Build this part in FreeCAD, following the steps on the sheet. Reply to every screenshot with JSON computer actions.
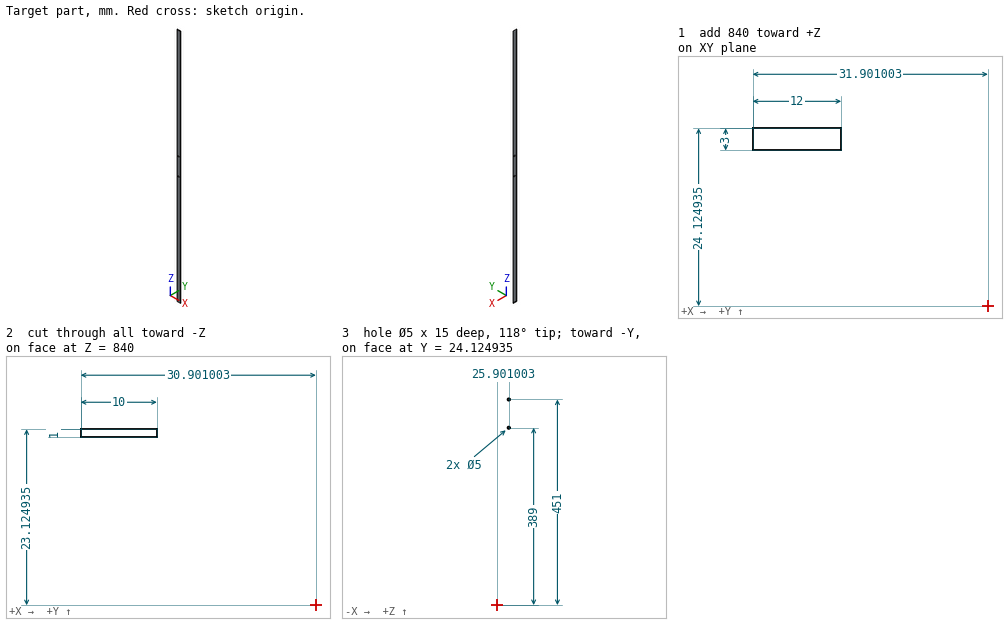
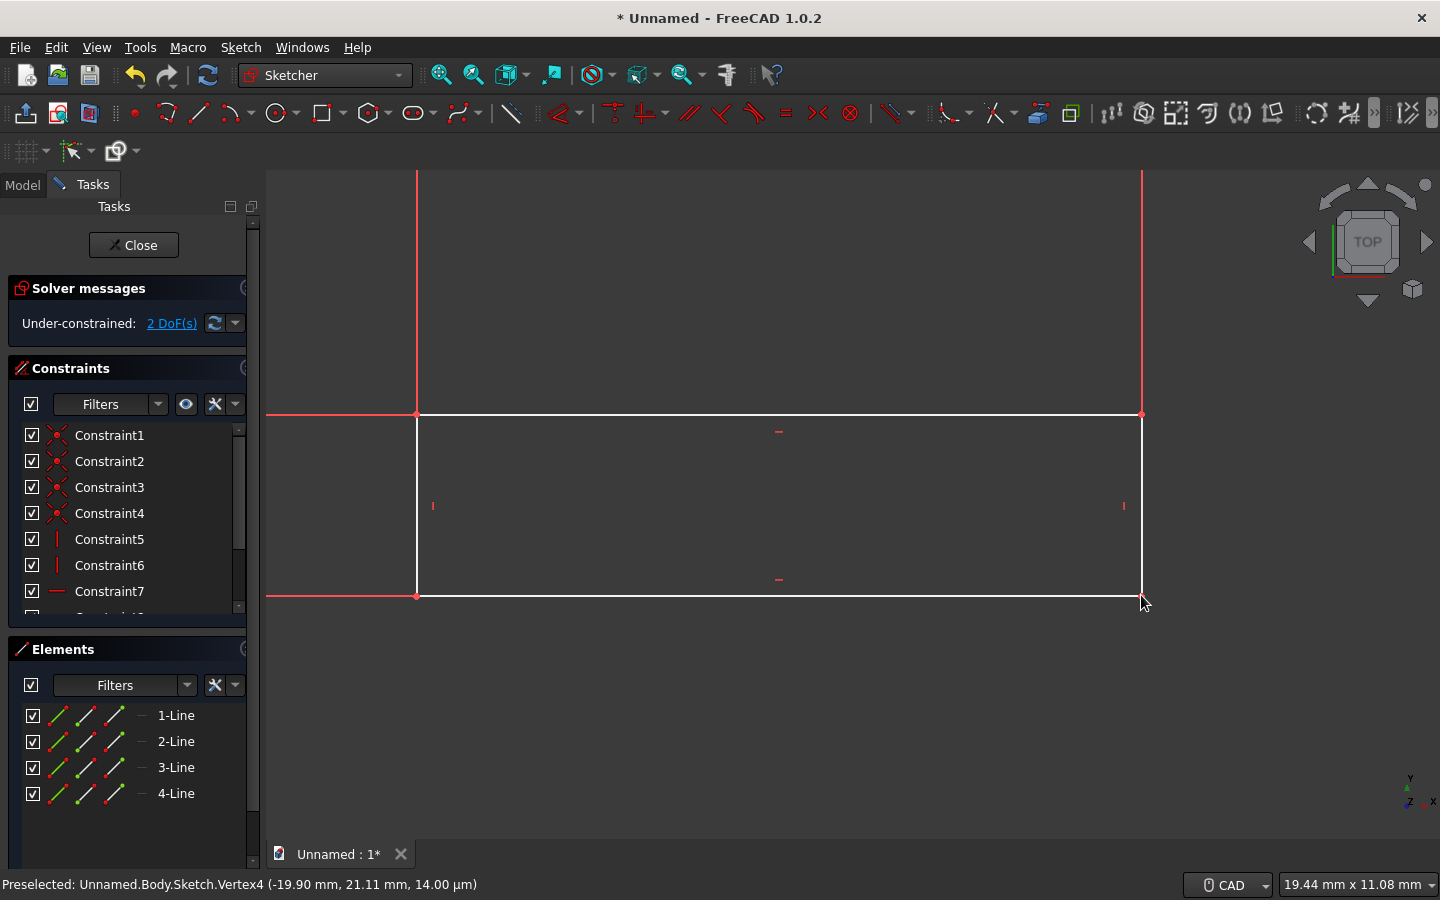
{"action": "left_click", "coordinate": [558, 114]}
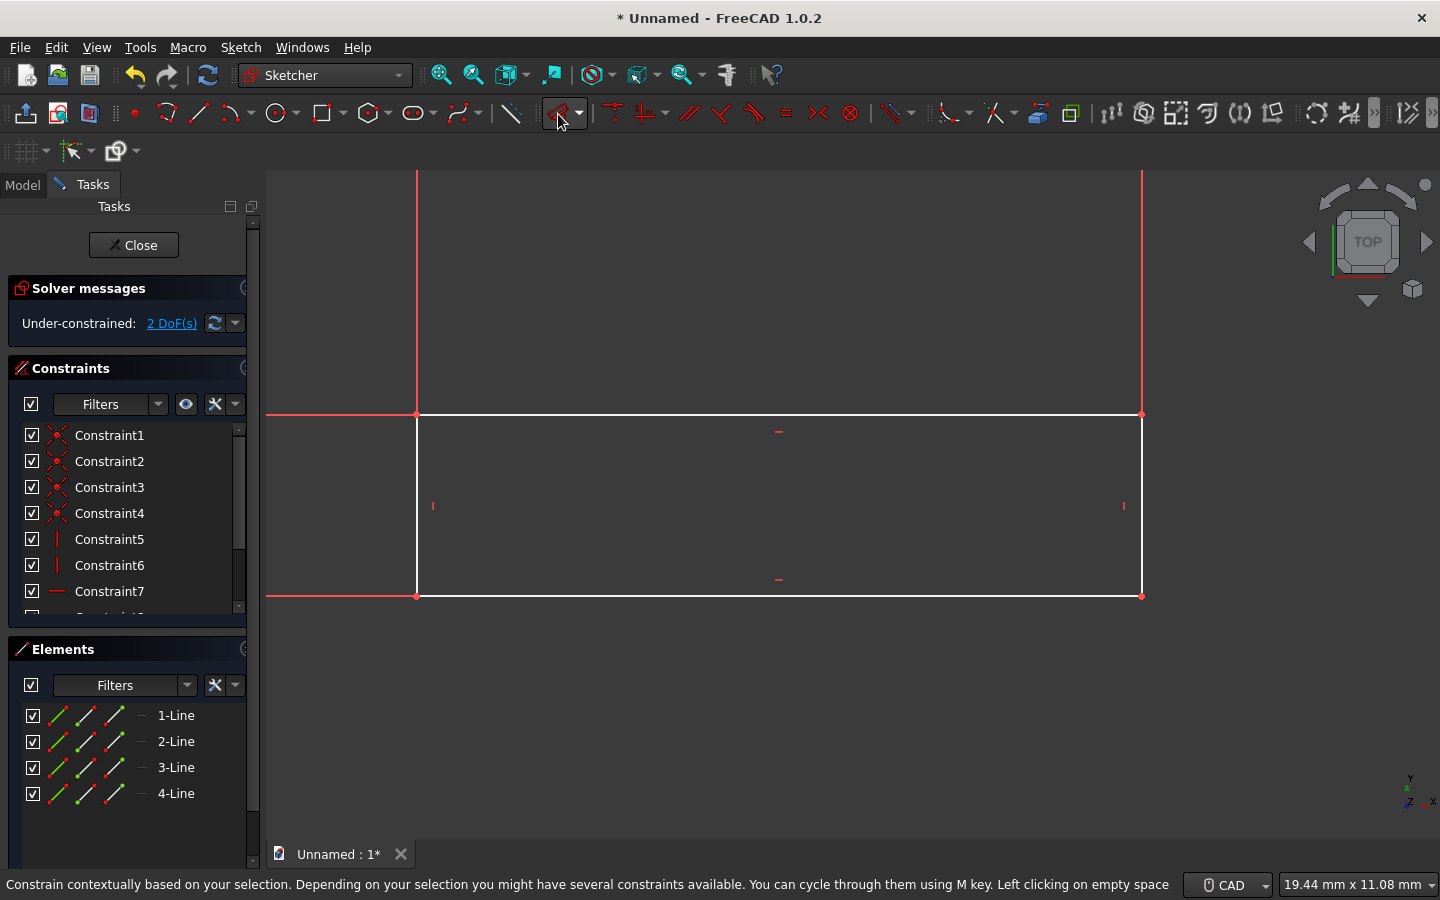
{"action": "left_click", "coordinate": [417, 415]}
{"action": "left_click", "coordinate": [846, 381]}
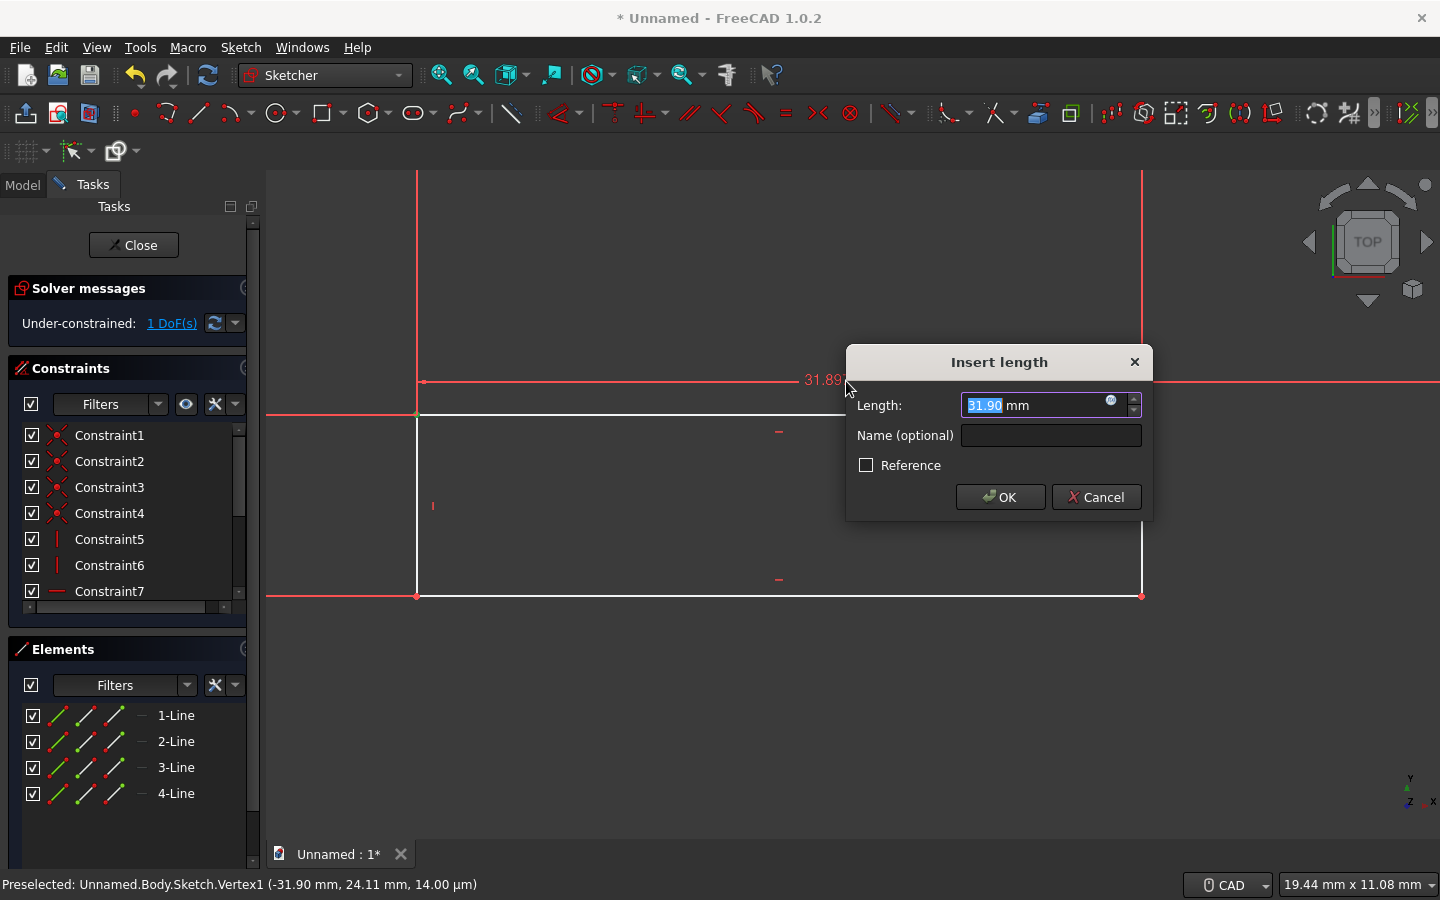
{"action": "type", "text": "31.901003"}
{"action": "key", "text": "Return"}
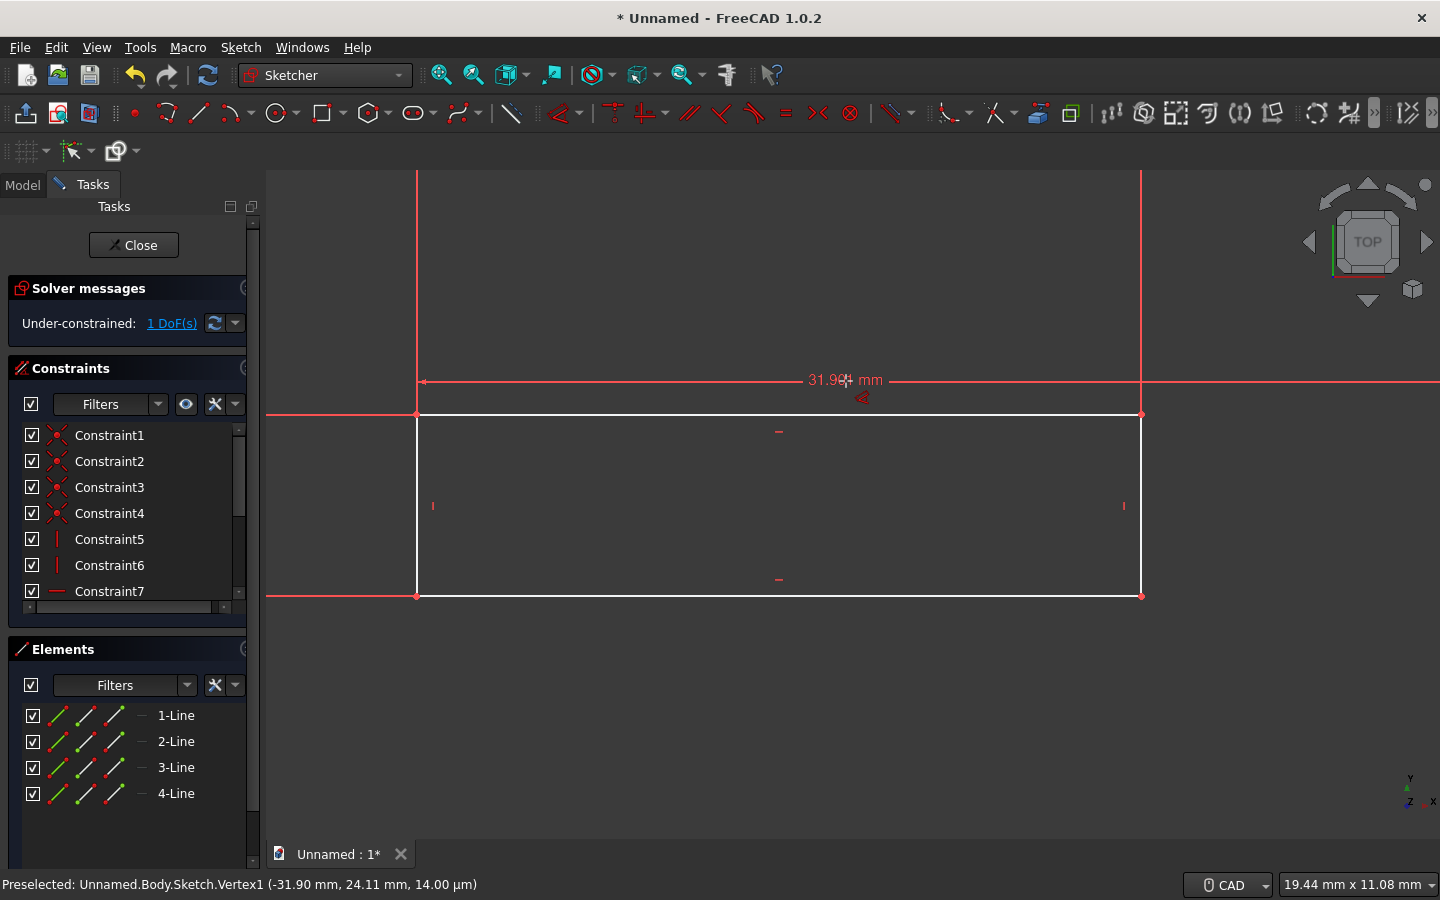
{"action": "left_click", "coordinate": [417, 415]}
{"action": "left_click", "coordinate": [383, 613]}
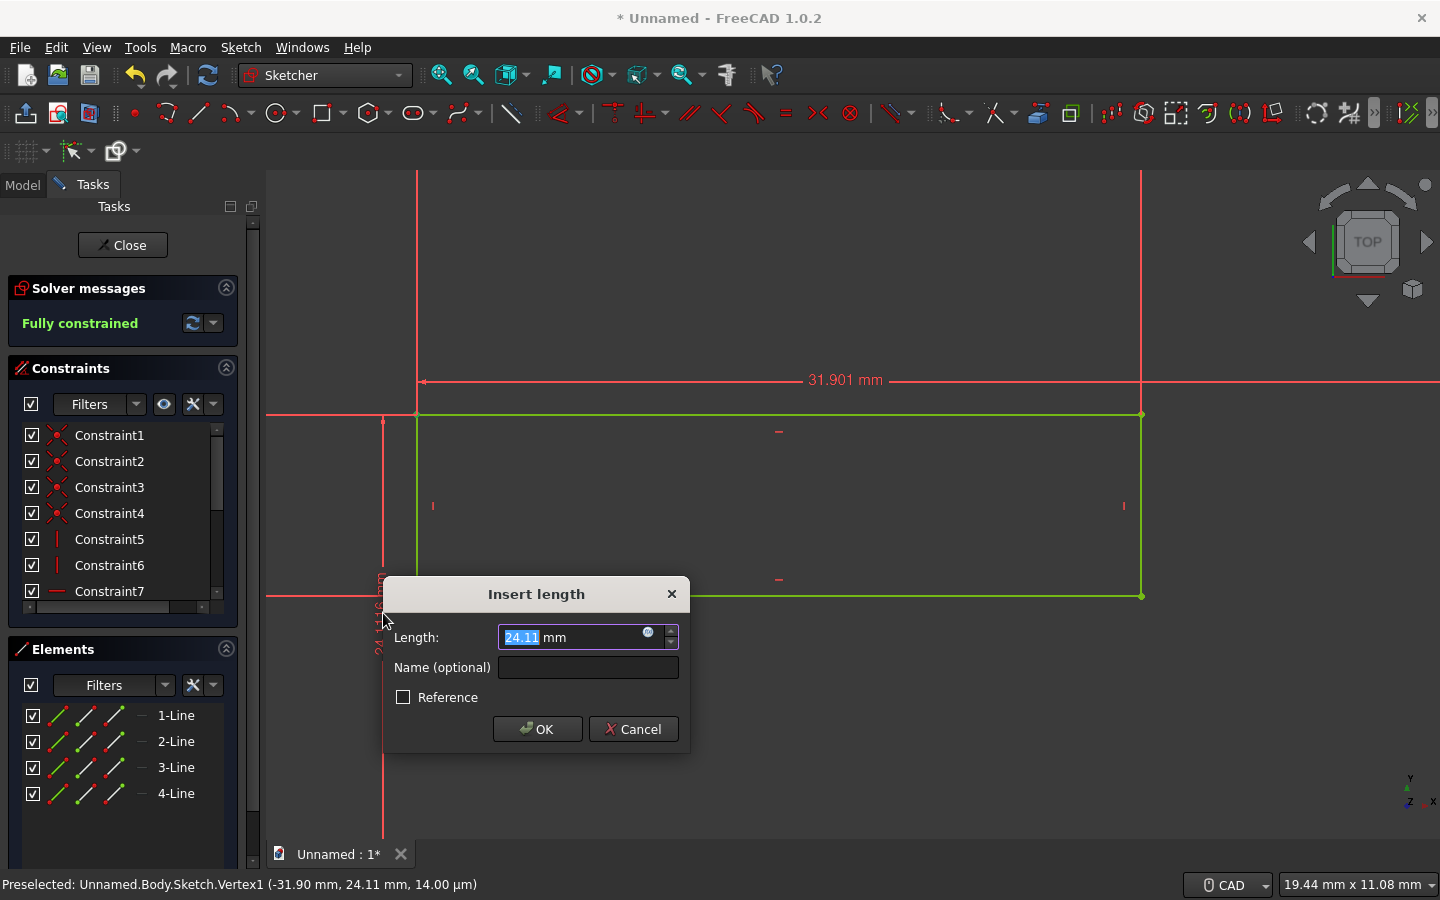
{"action": "type", "text": "24.124935"}
{"action": "key", "text": "Return"}
{"action": "key", "text": "Escape"}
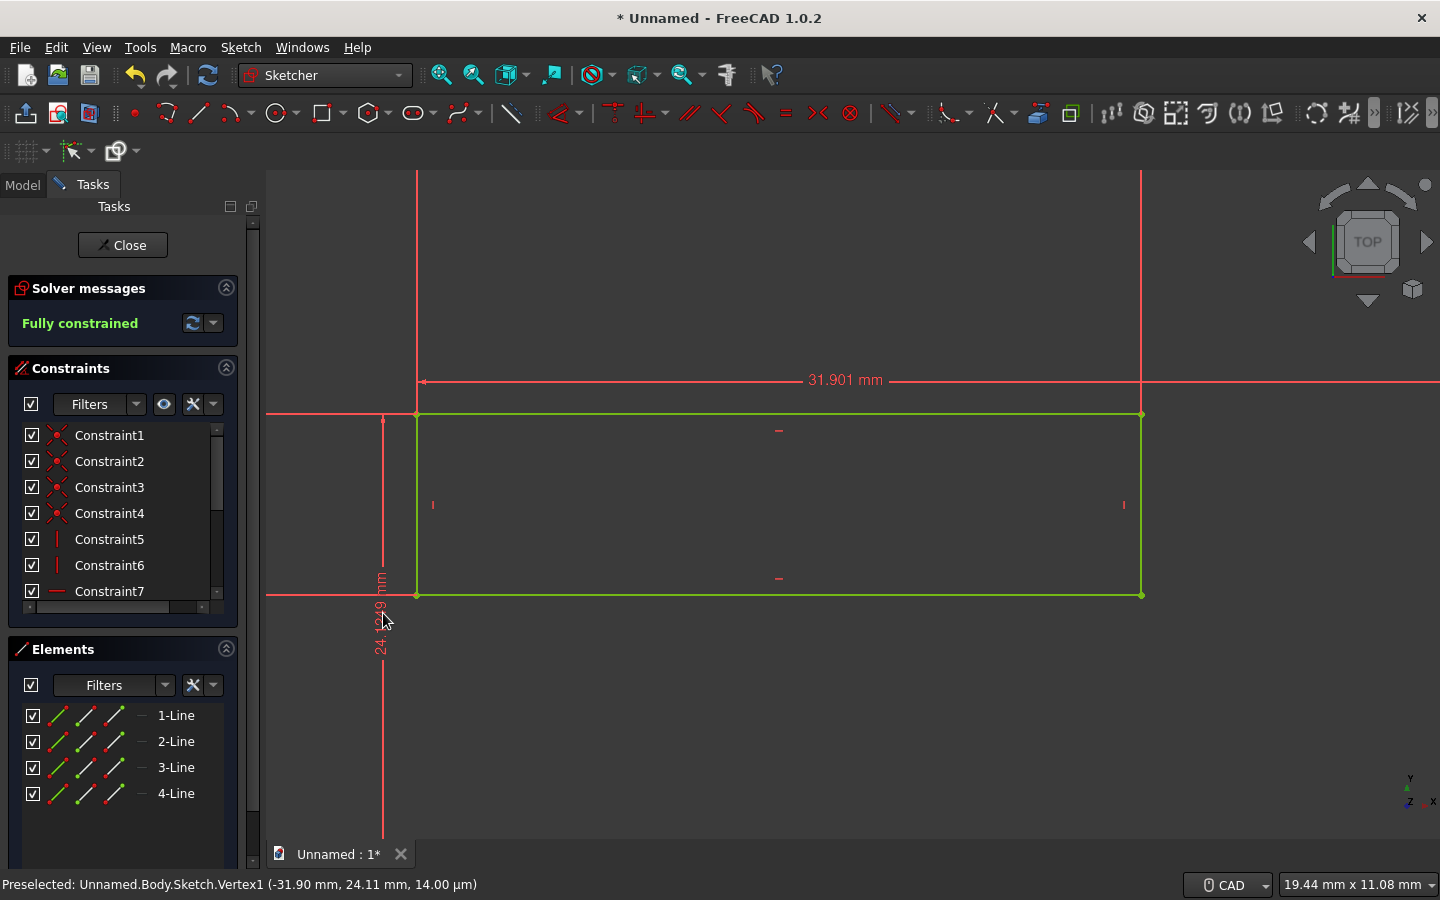
{"action": "left_click", "coordinate": [123, 245]}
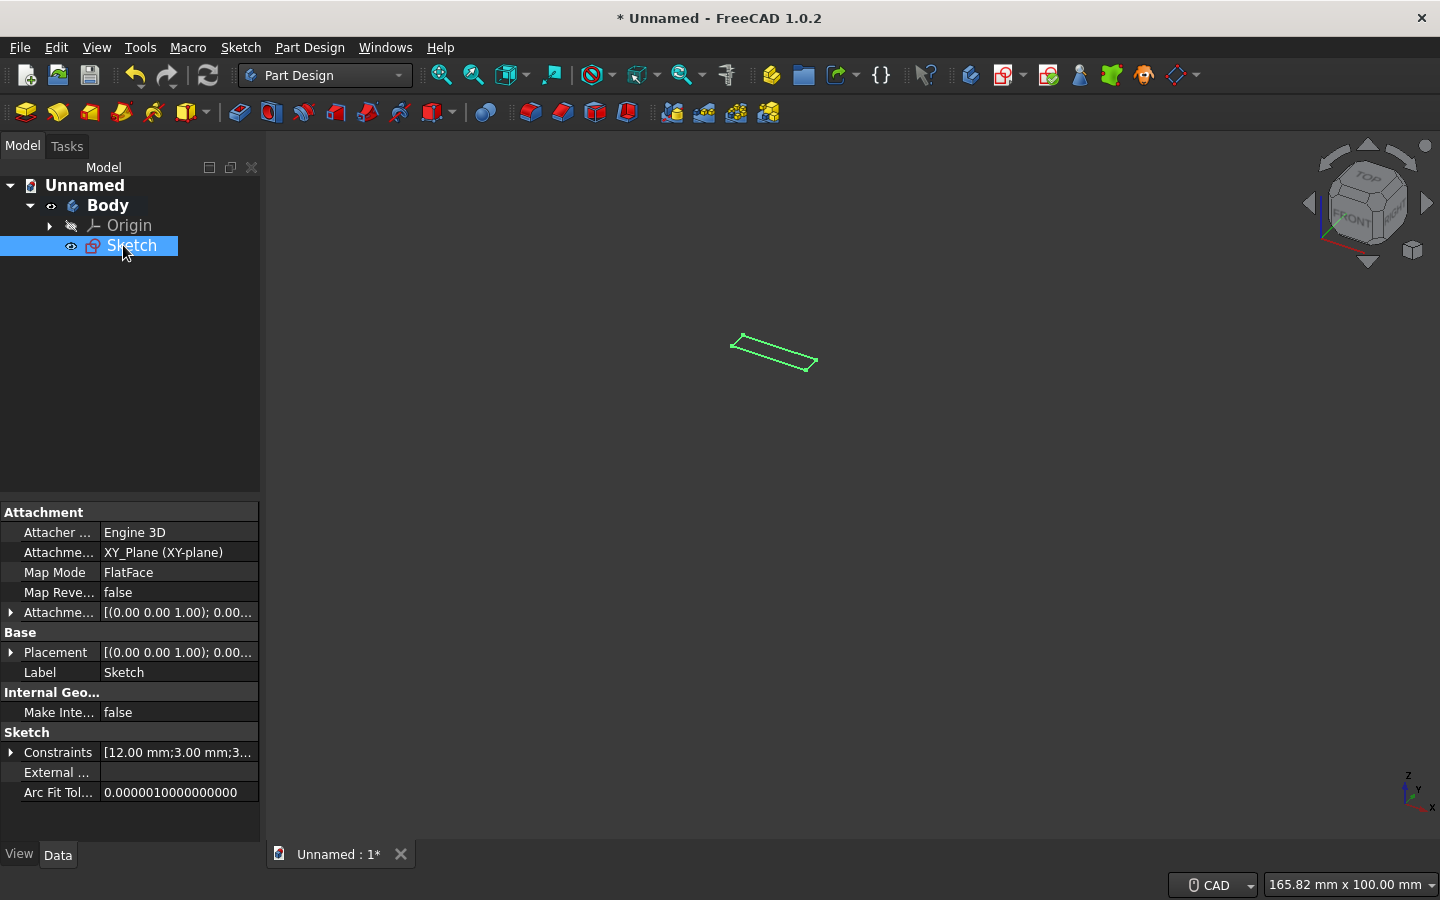
{"action": "left_click", "coordinate": [26, 112]}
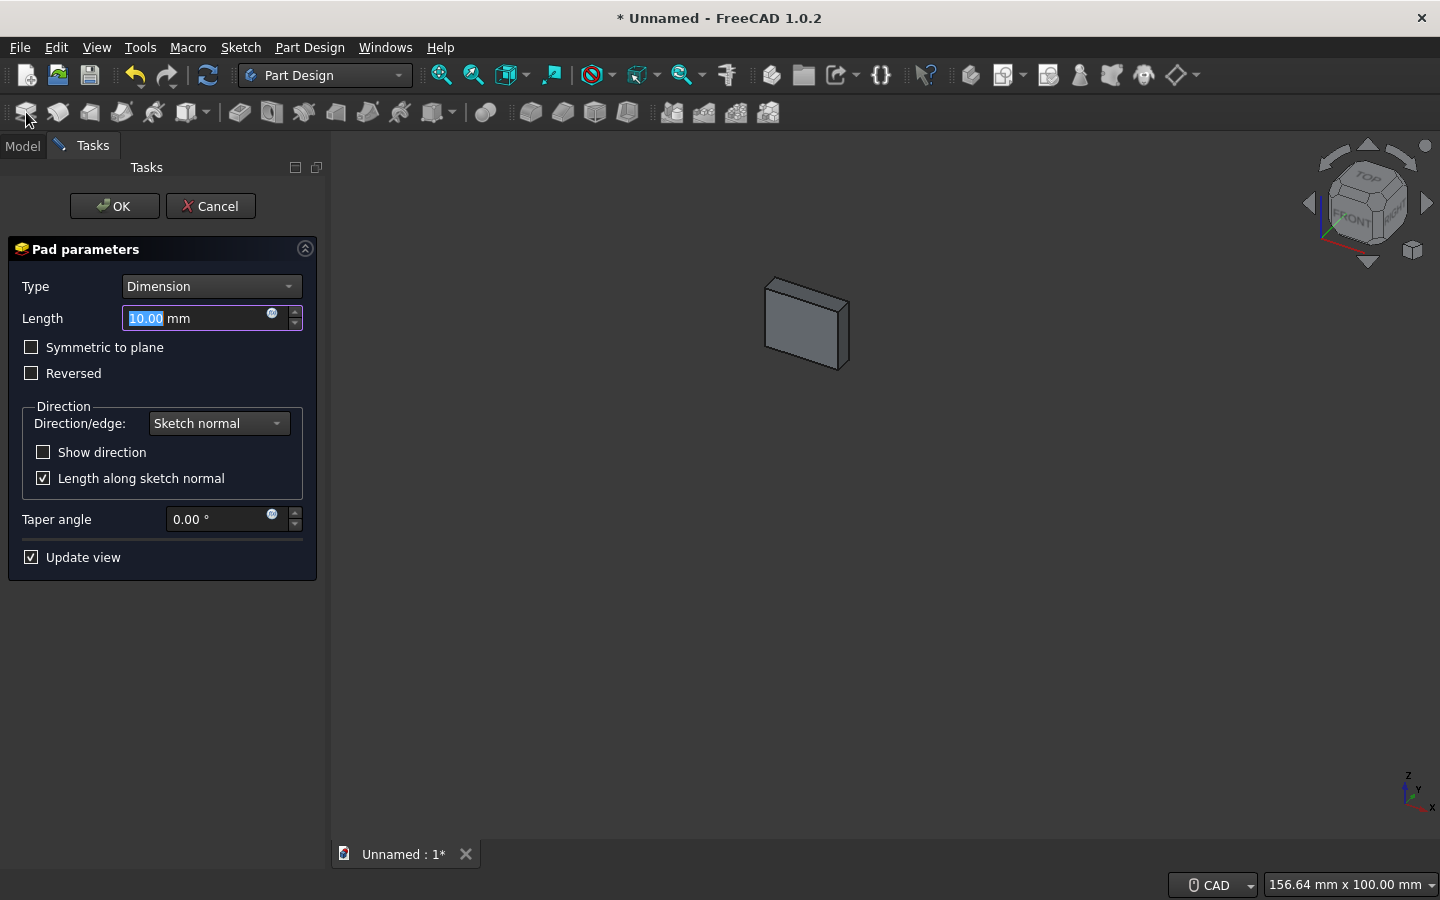
{"action": "type", "text": "840"}
{"action": "key", "text": "Tab"}